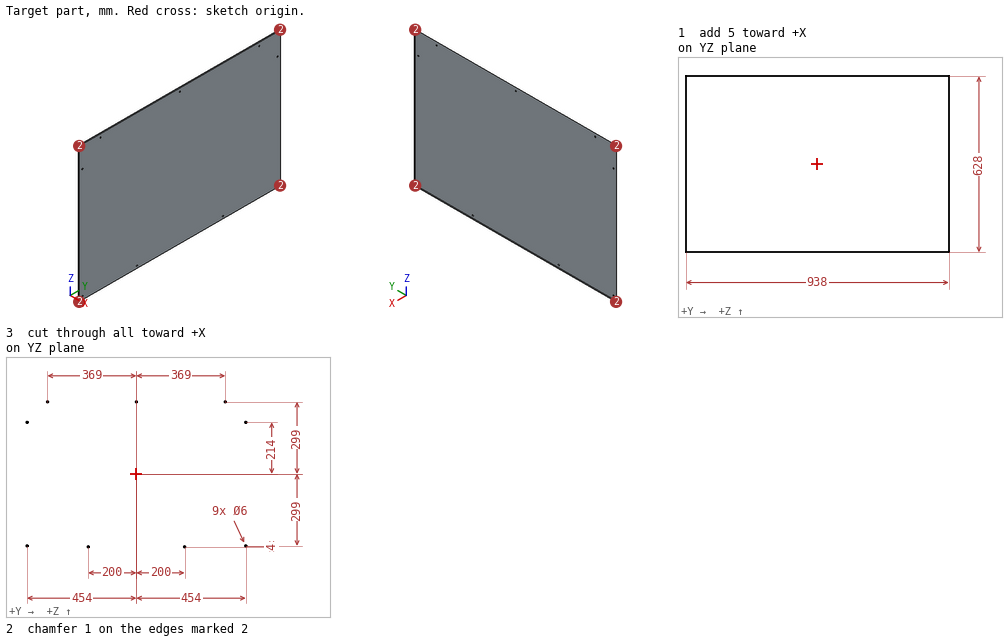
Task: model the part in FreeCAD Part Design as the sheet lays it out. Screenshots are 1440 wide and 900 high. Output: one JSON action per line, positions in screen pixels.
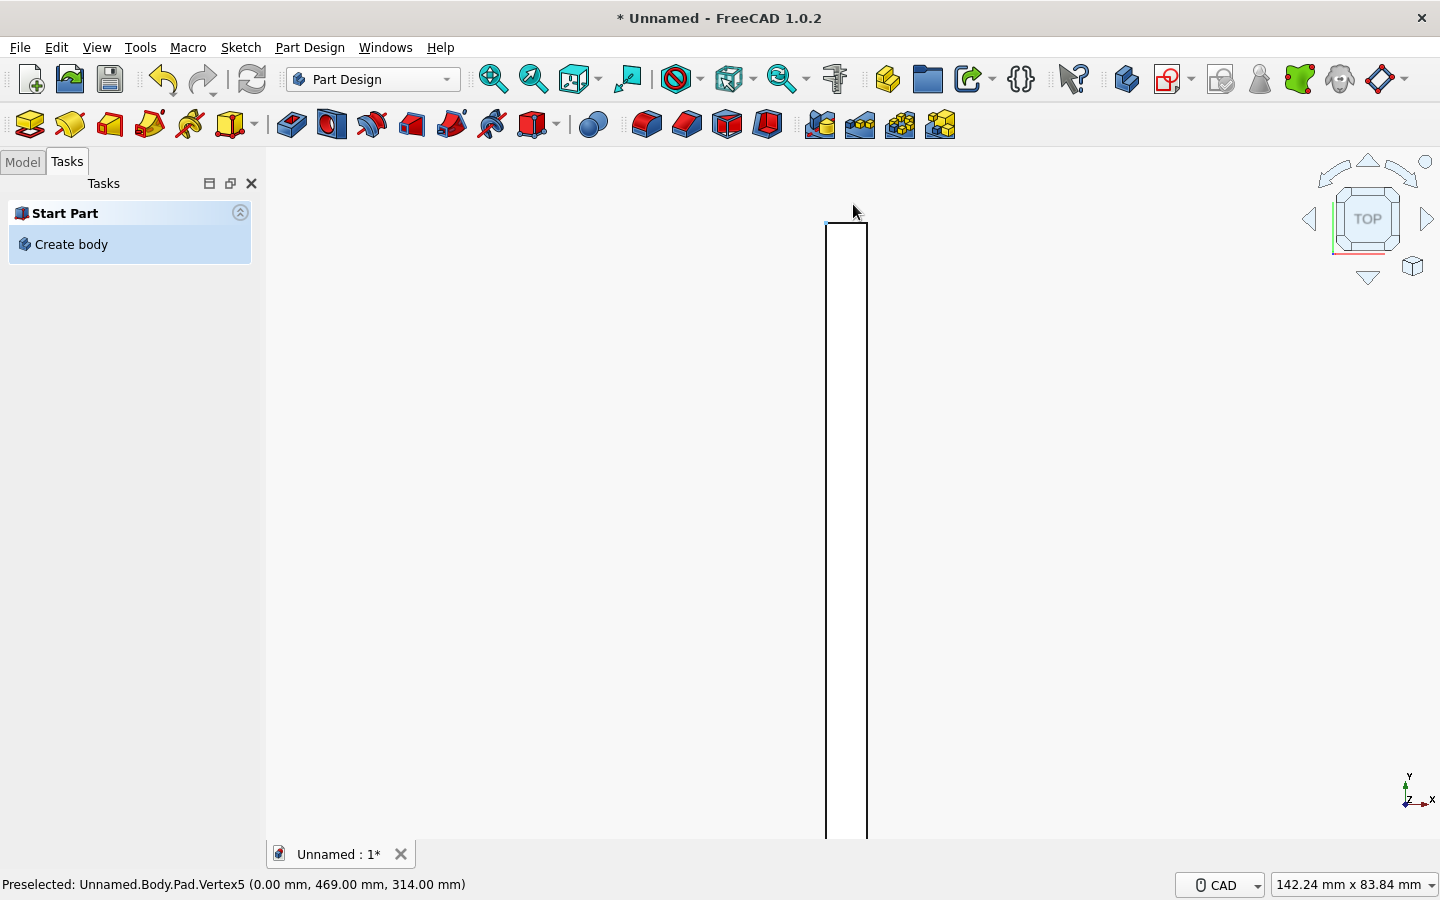
{"action": "left_click", "coordinate": [847, 222]}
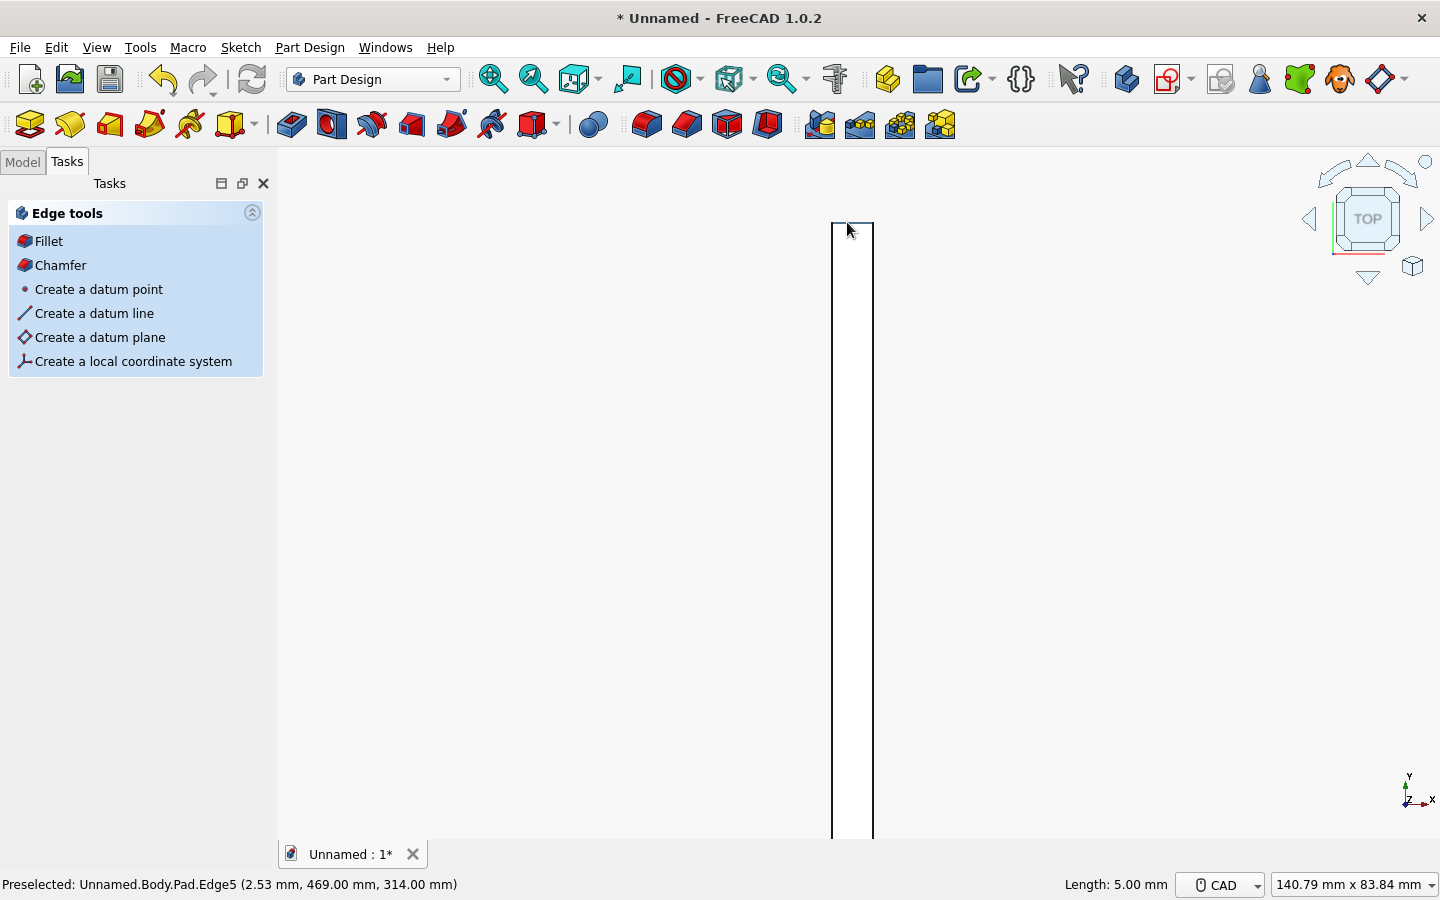
{"action": "key", "text": "v f"}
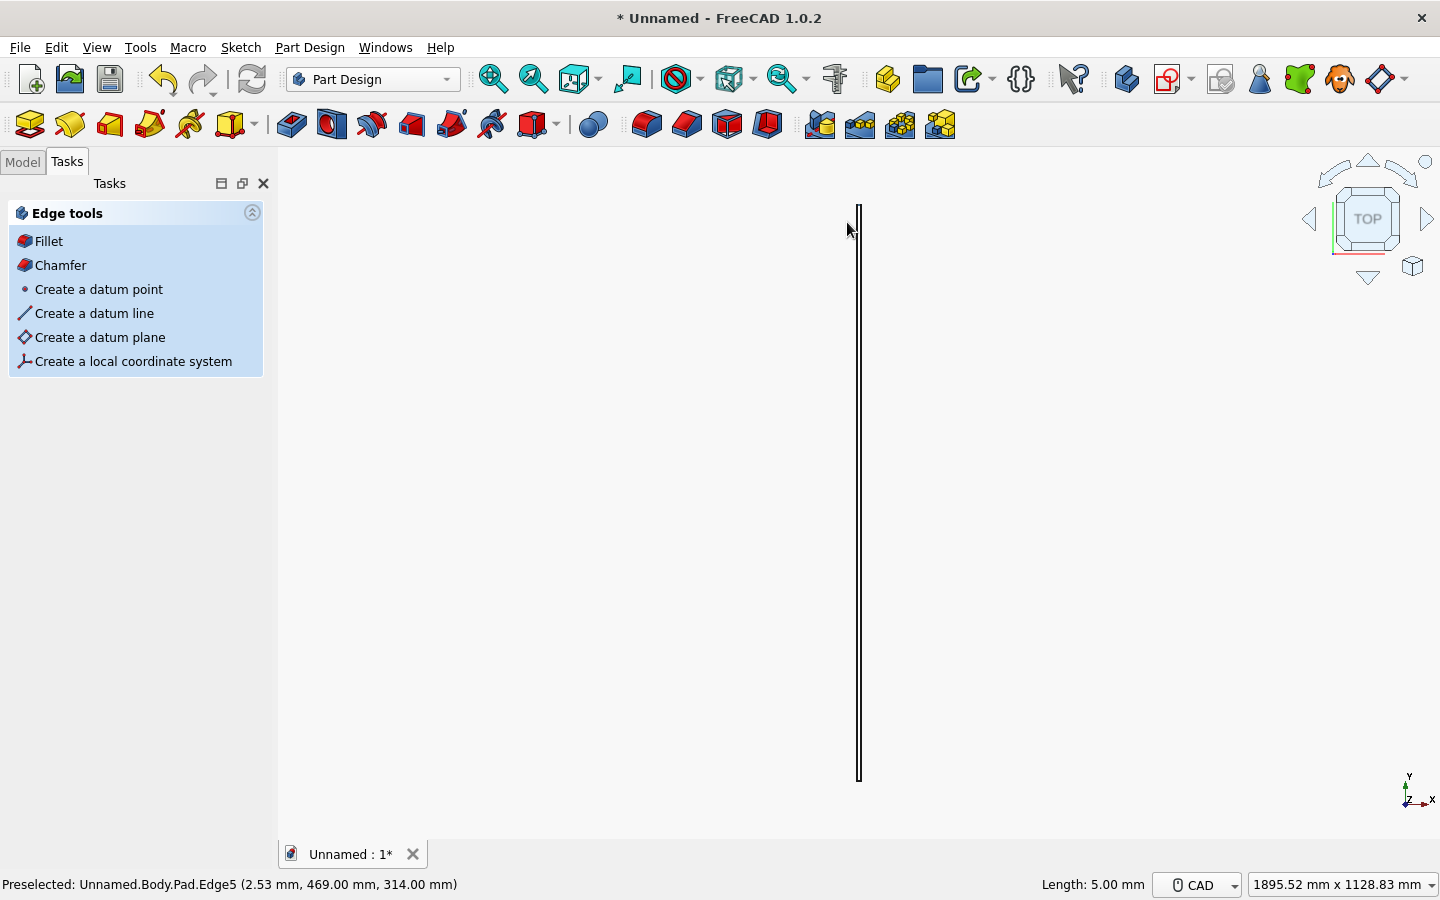
{"action": "key", "text": "1"}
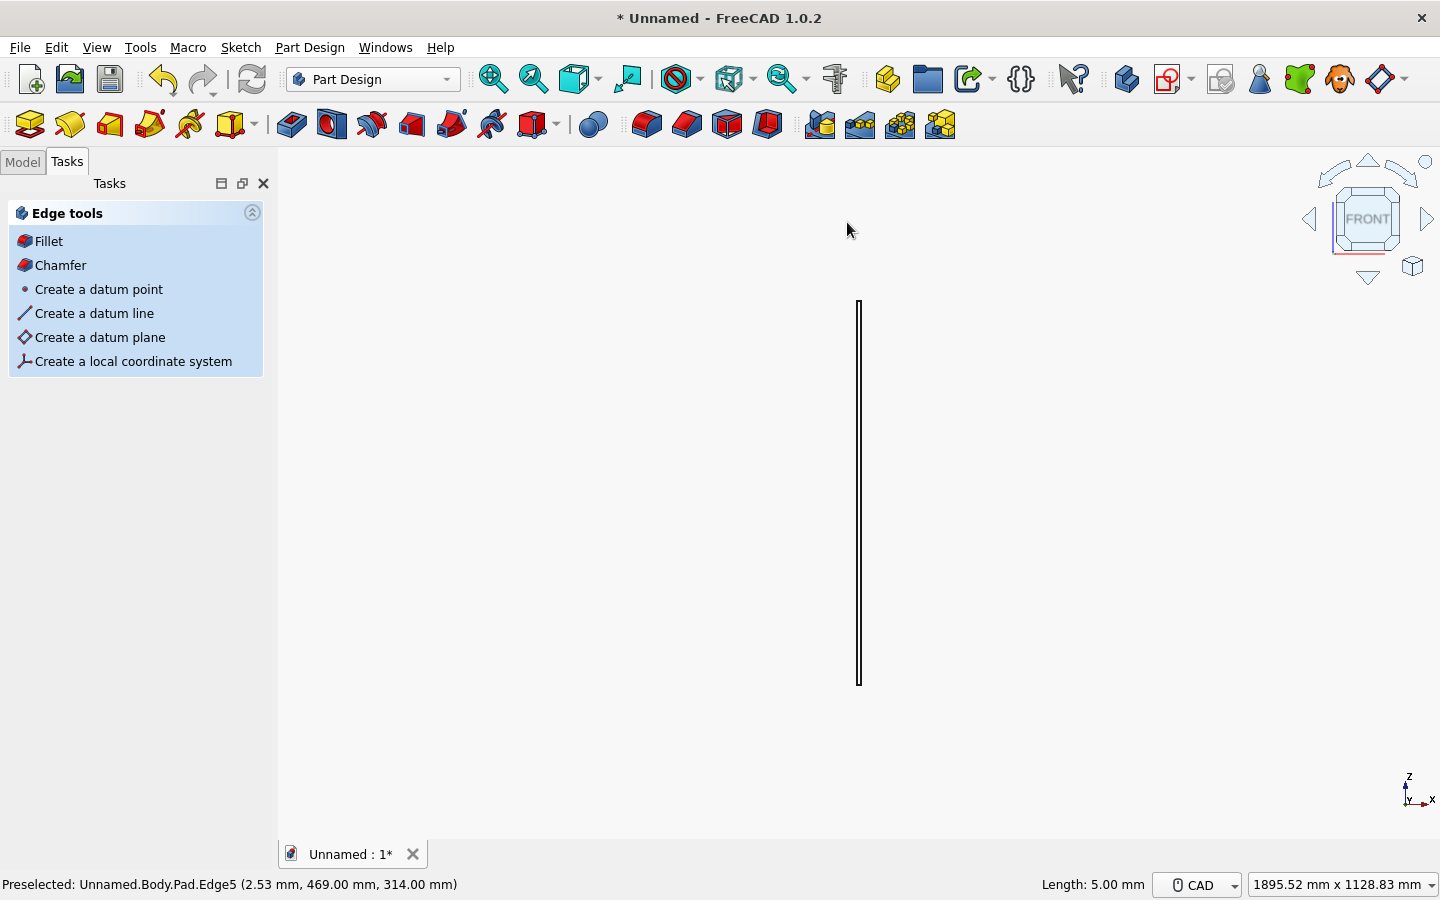
{"action": "scroll", "coordinate": [859, 684], "scroll_direction": "up", "scroll_amount": 13}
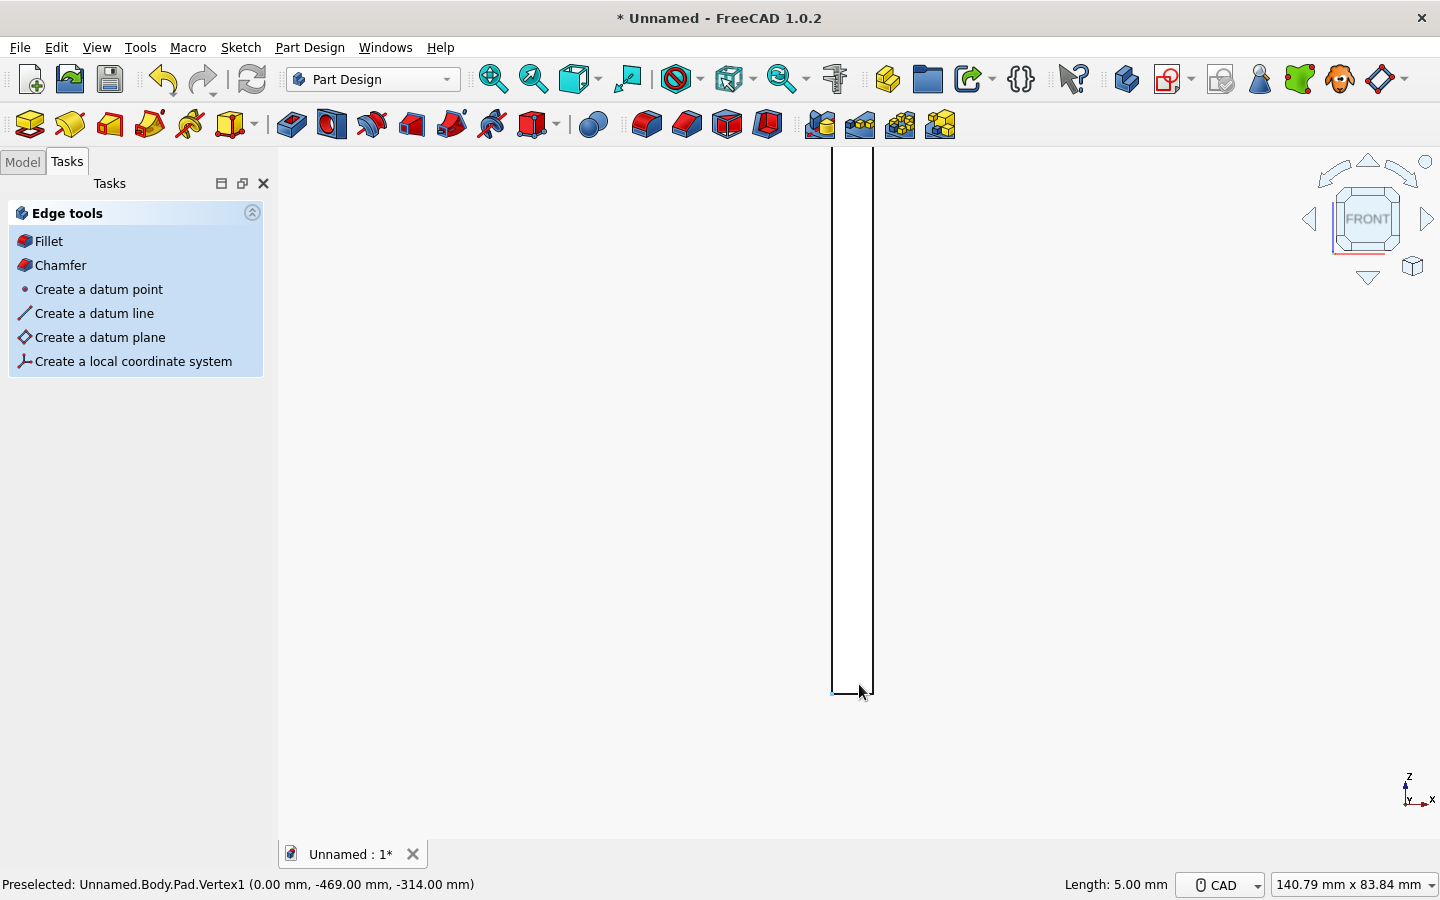
{"action": "left_click", "coordinate": [853, 693], "text": "ctrl"}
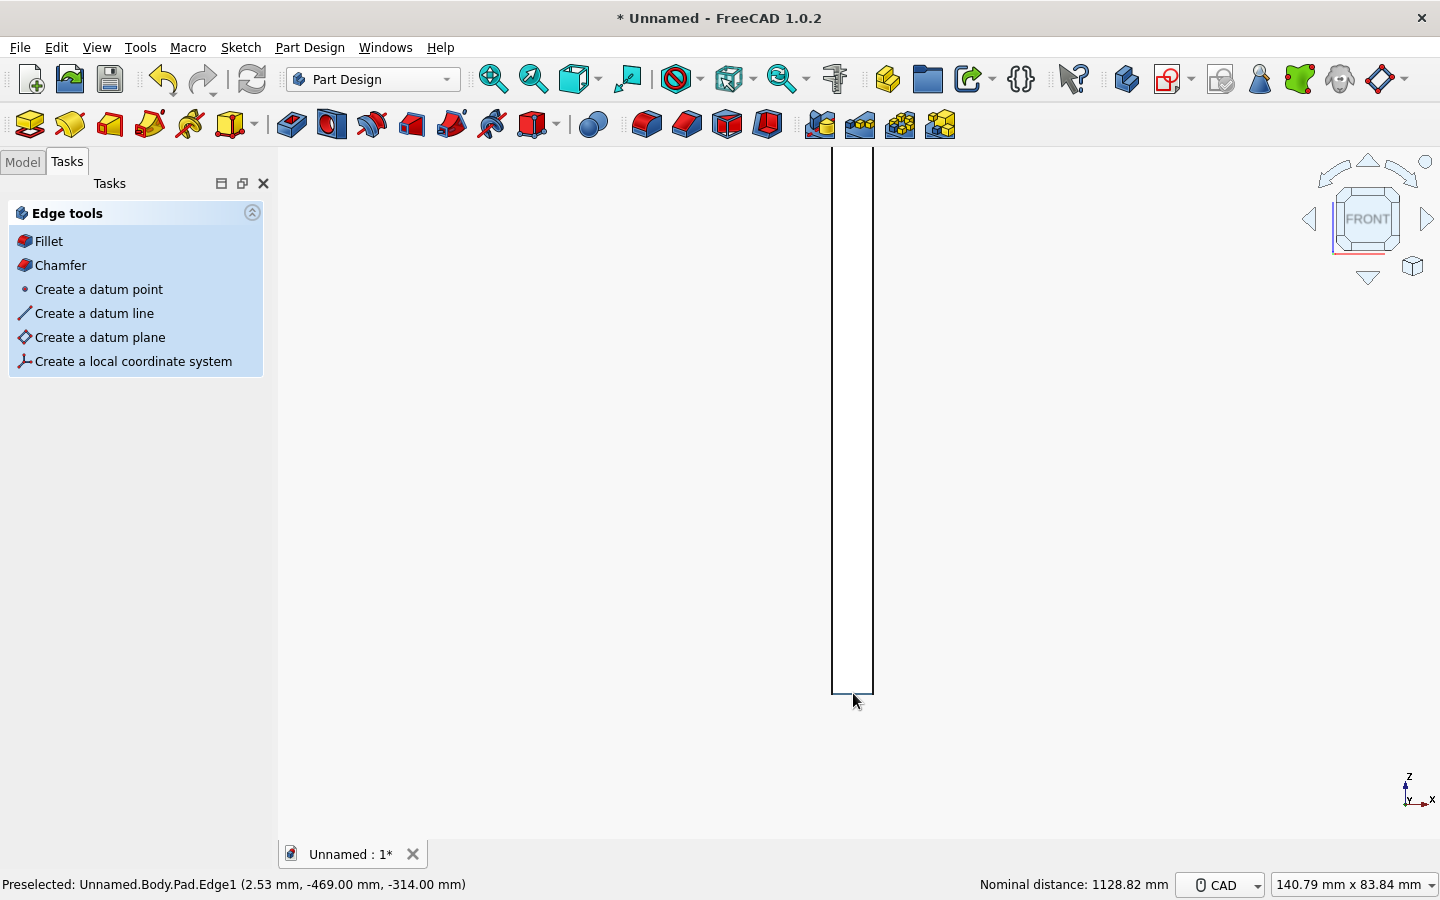
{"action": "key", "text": "v f"}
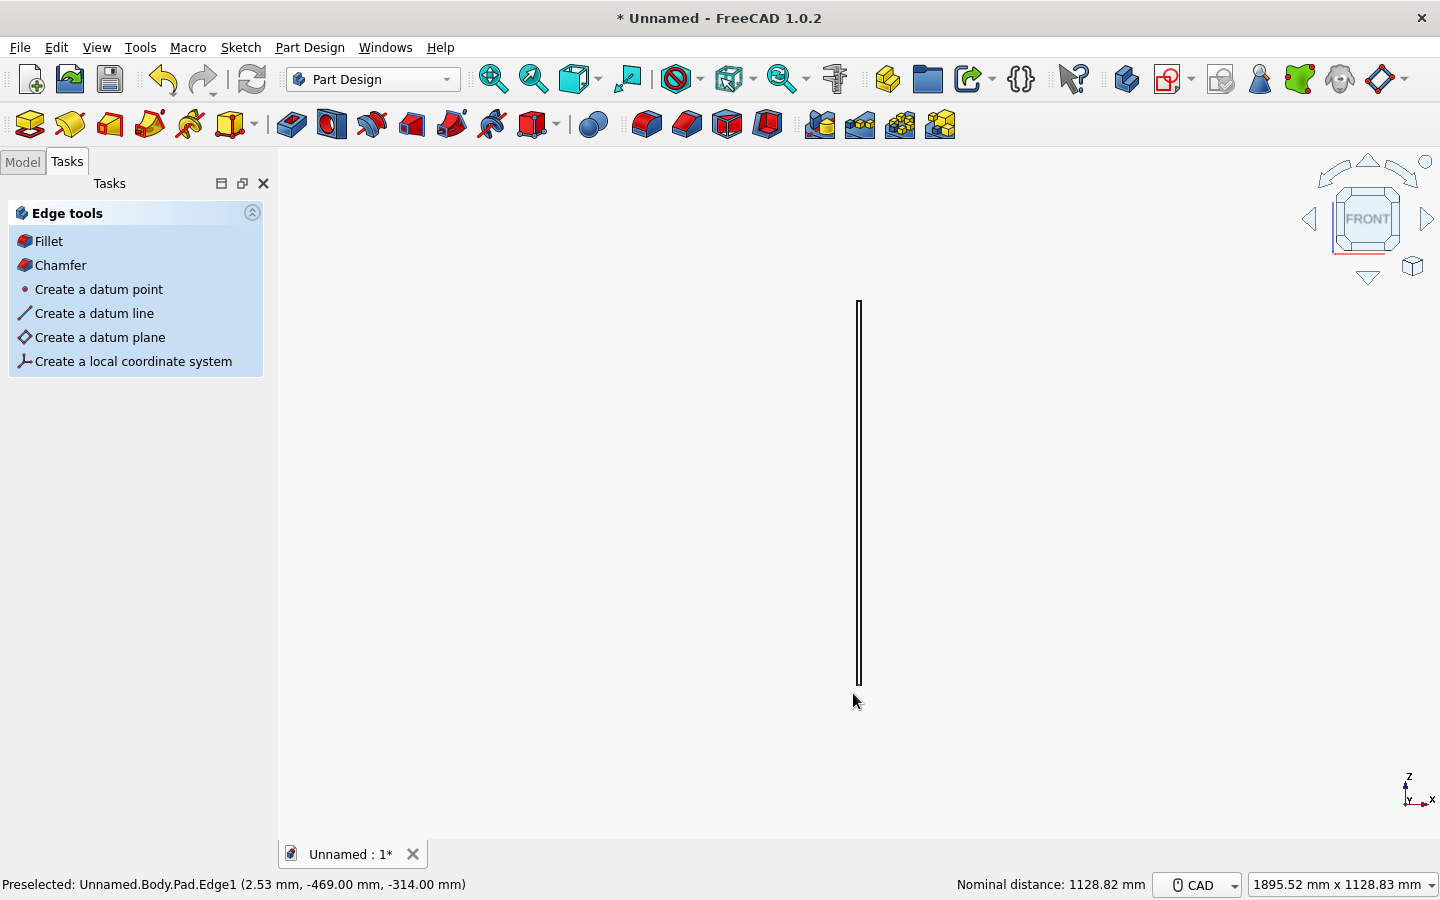
{"action": "key", "text": "3"}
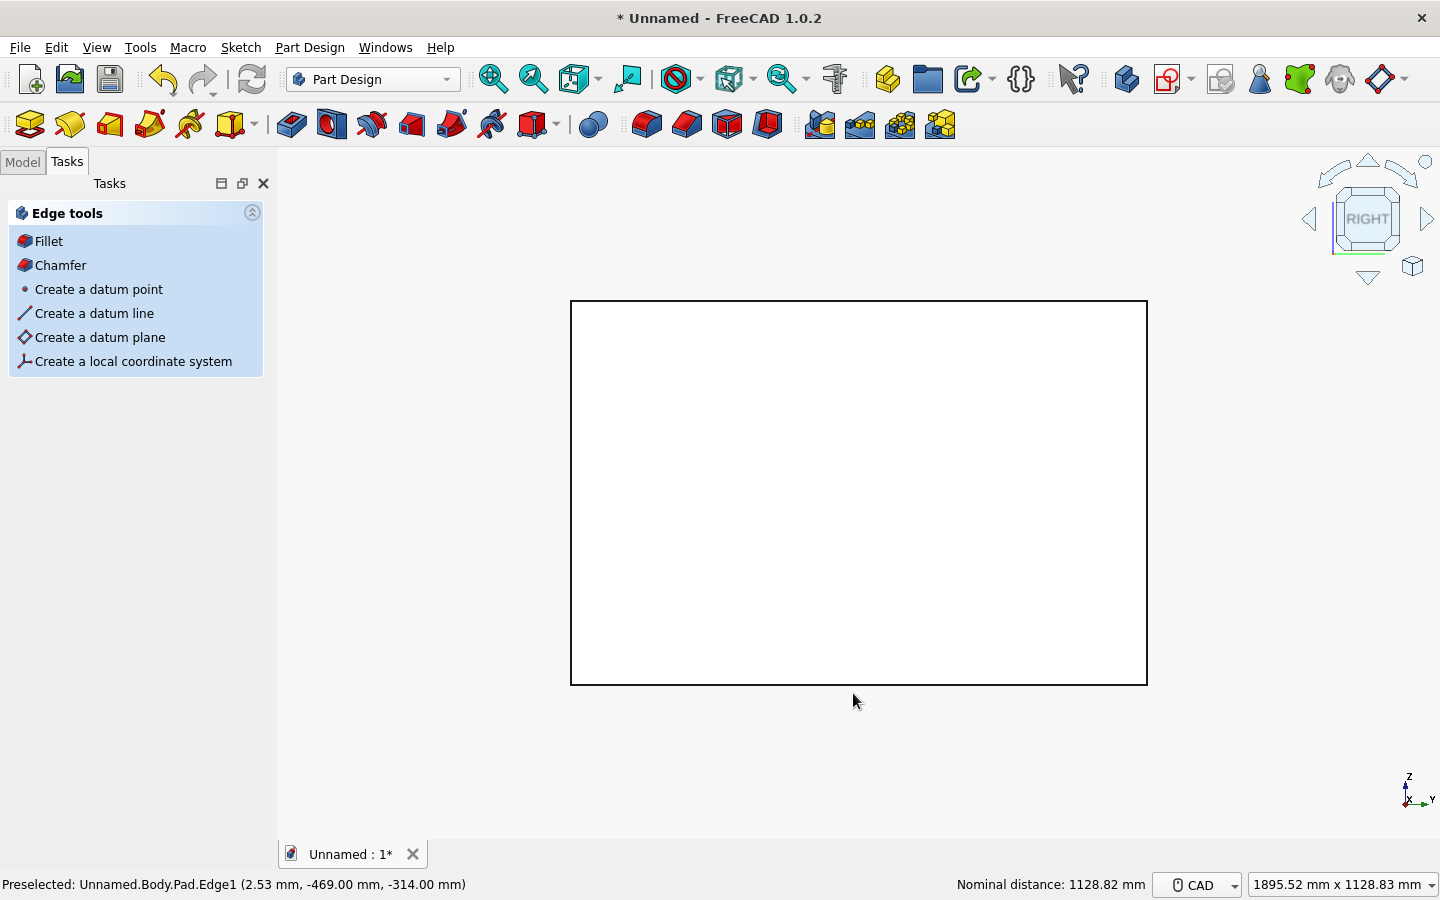
{"action": "scroll", "coordinate": [1147, 684], "scroll_direction": "up", "scroll_amount": 13}